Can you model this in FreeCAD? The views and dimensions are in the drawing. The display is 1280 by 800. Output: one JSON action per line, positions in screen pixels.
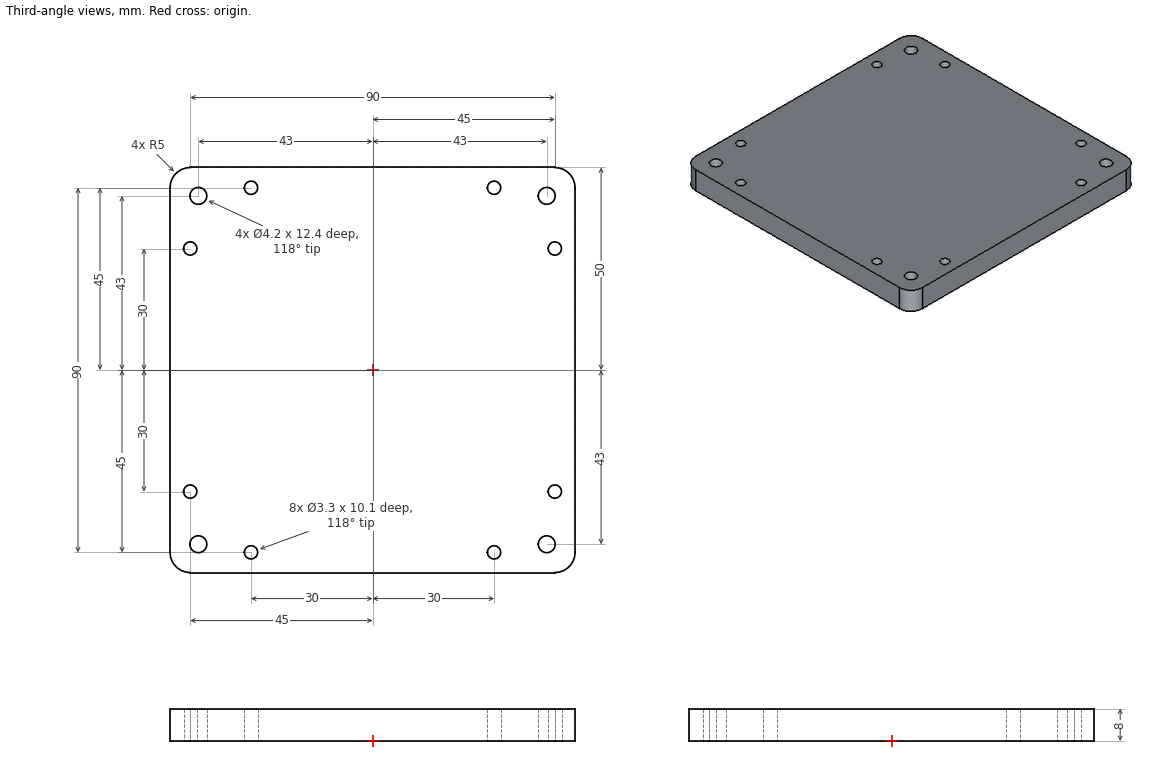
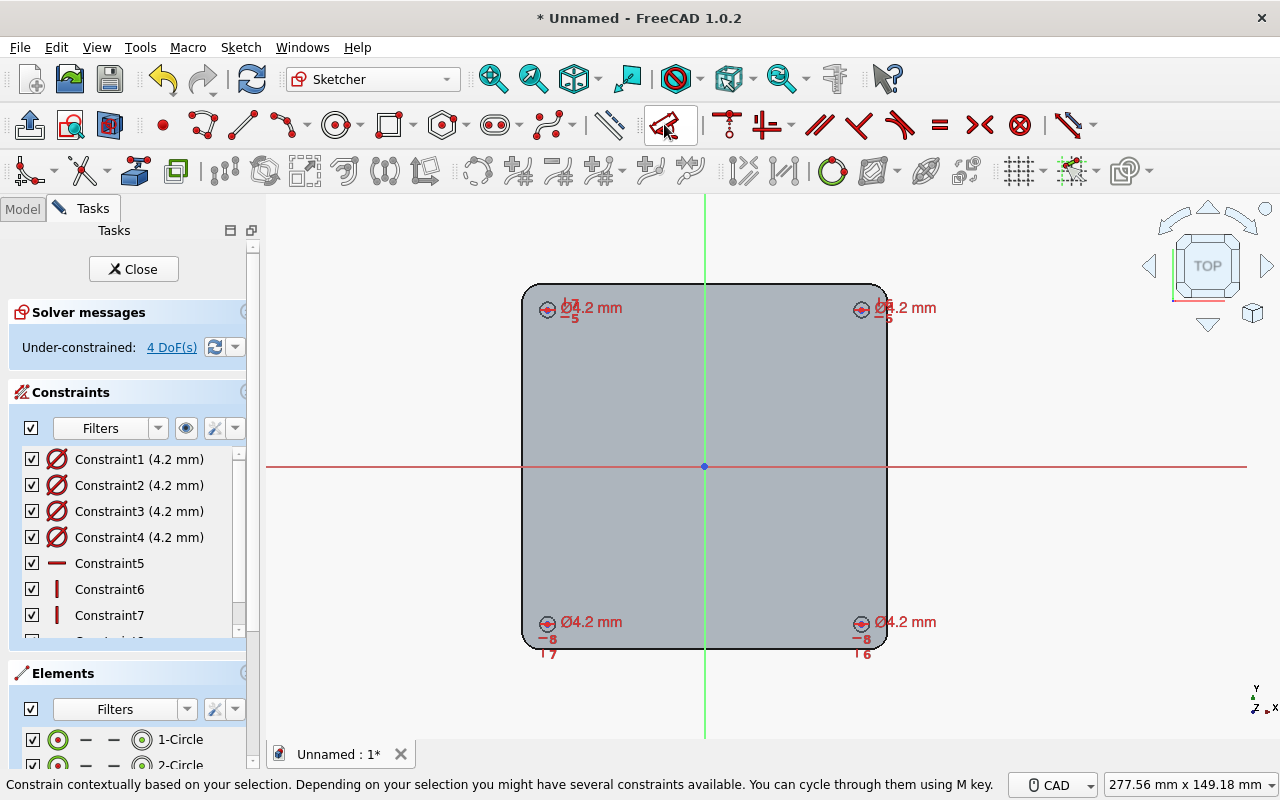
{"action": "left_click", "coordinate": [548, 310]}
{"action": "left_click", "coordinate": [626, 276]}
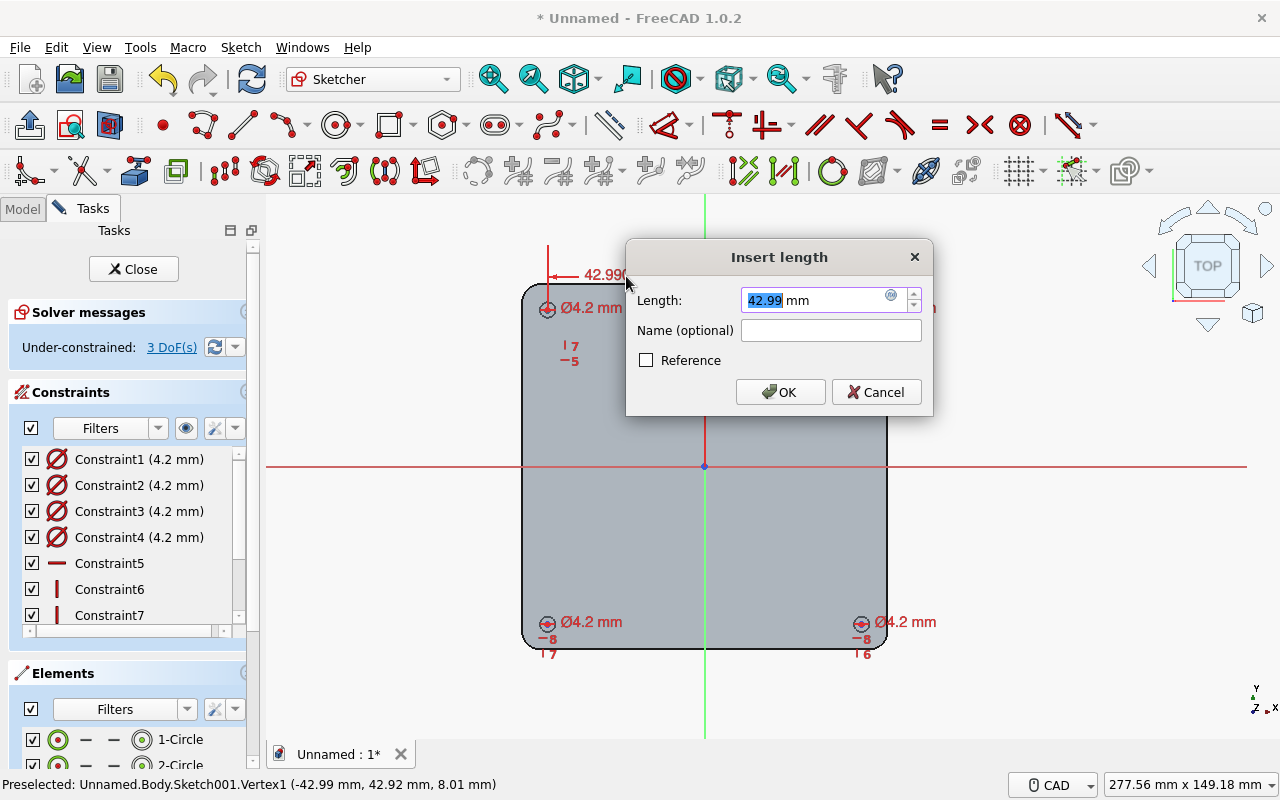
{"action": "type", "text": "43"}
{"action": "key", "text": "Return"}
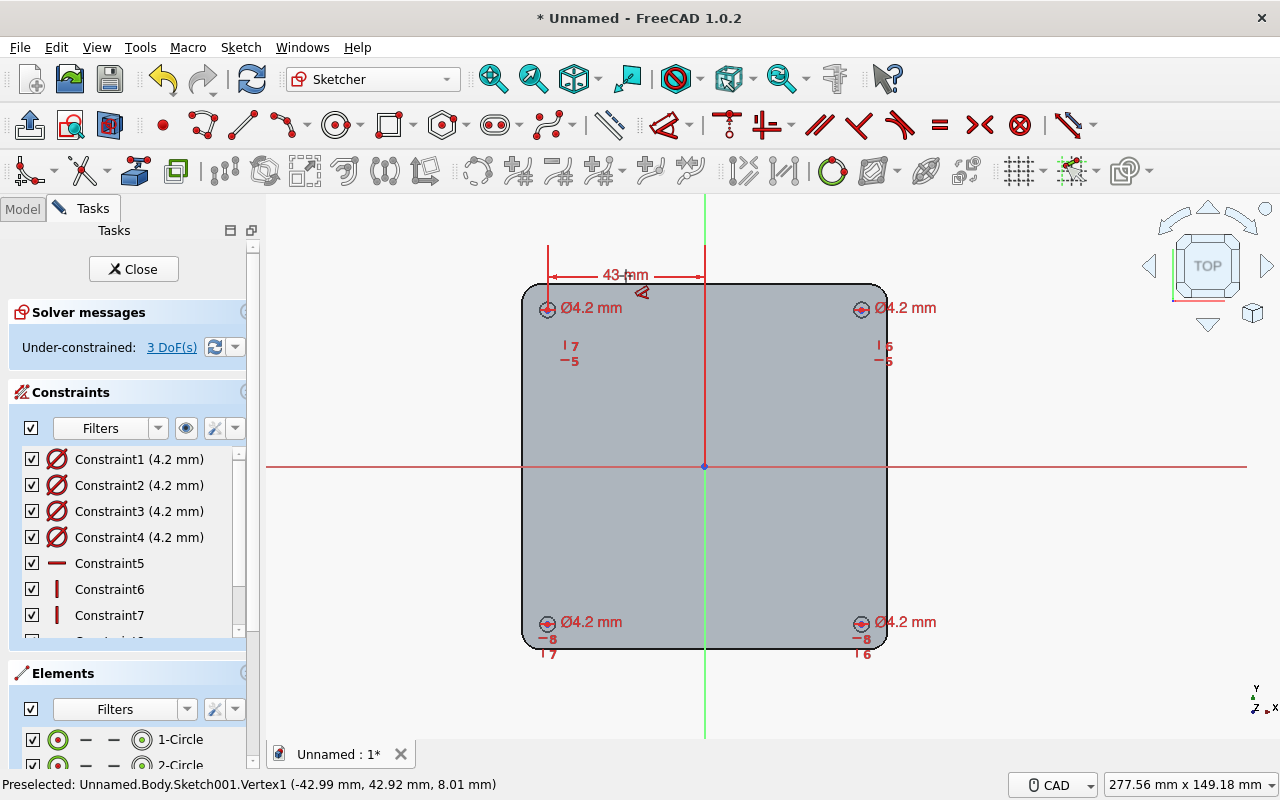
{"action": "left_click", "coordinate": [548, 310]}
{"action": "left_click", "coordinate": [514, 388]}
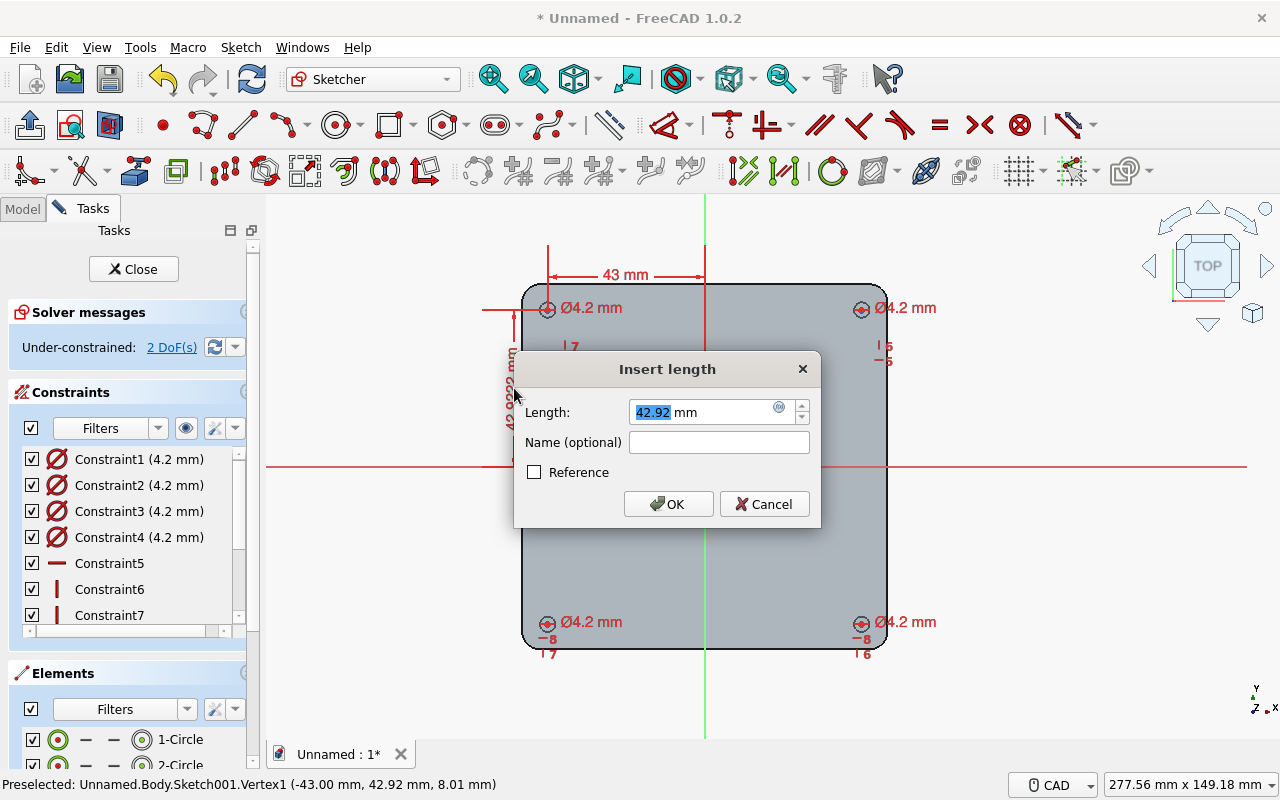
{"action": "type", "text": "43"}
{"action": "key", "text": "Return"}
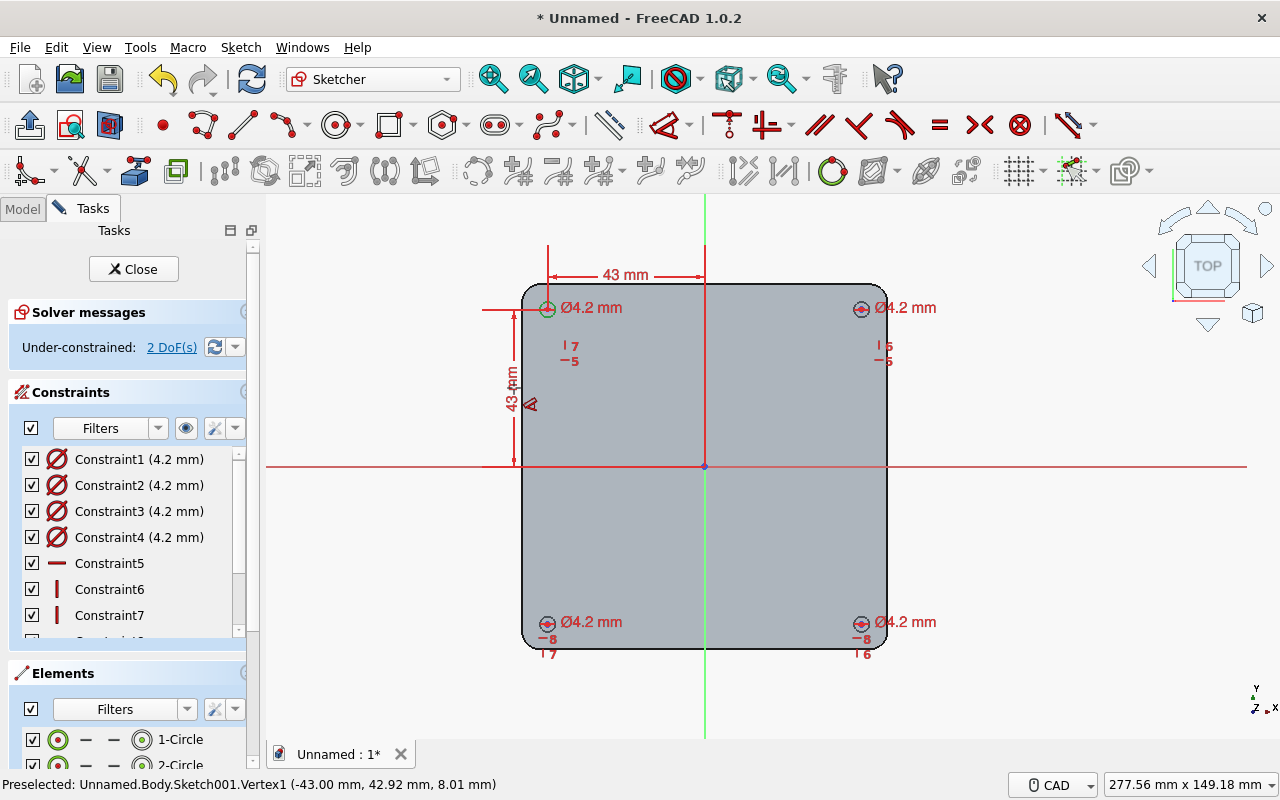
{"action": "left_click", "coordinate": [862, 310]}
{"action": "left_click", "coordinate": [783, 276]}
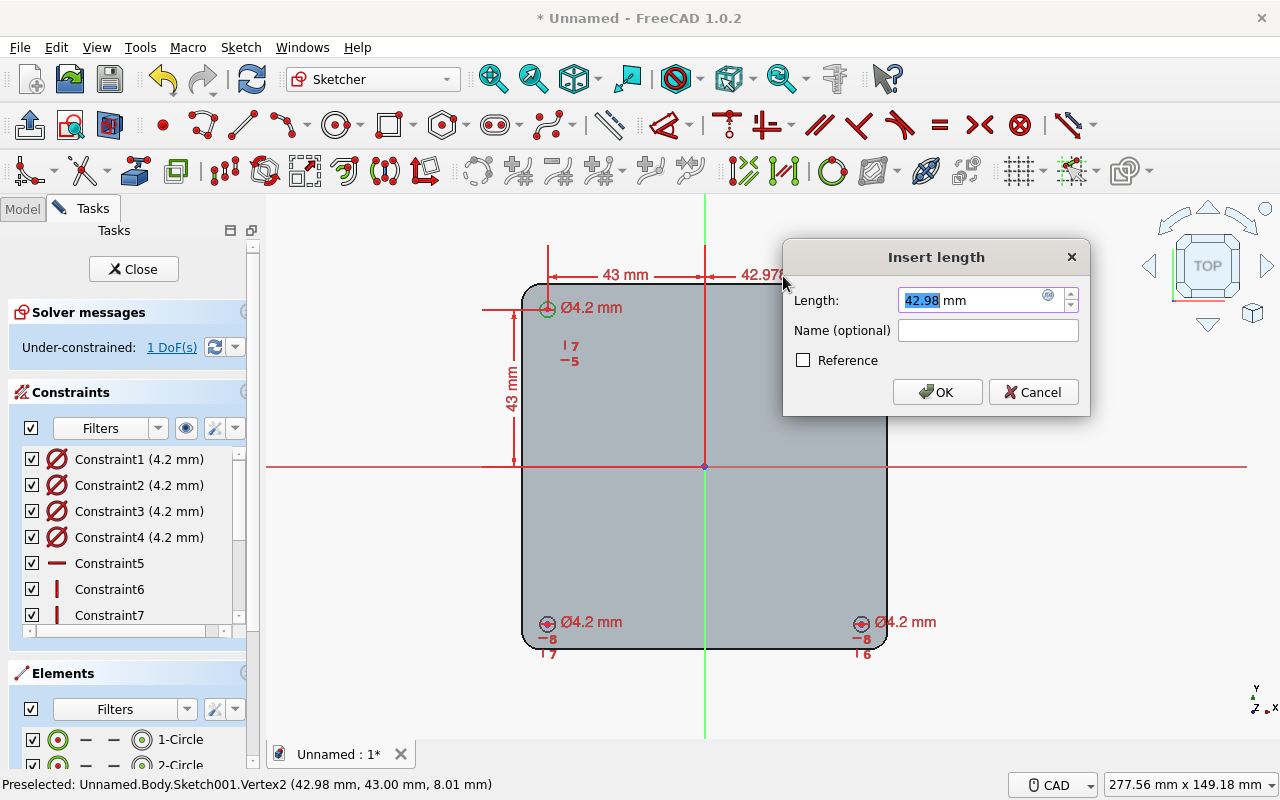
{"action": "type", "text": "43"}
{"action": "key", "text": "Return"}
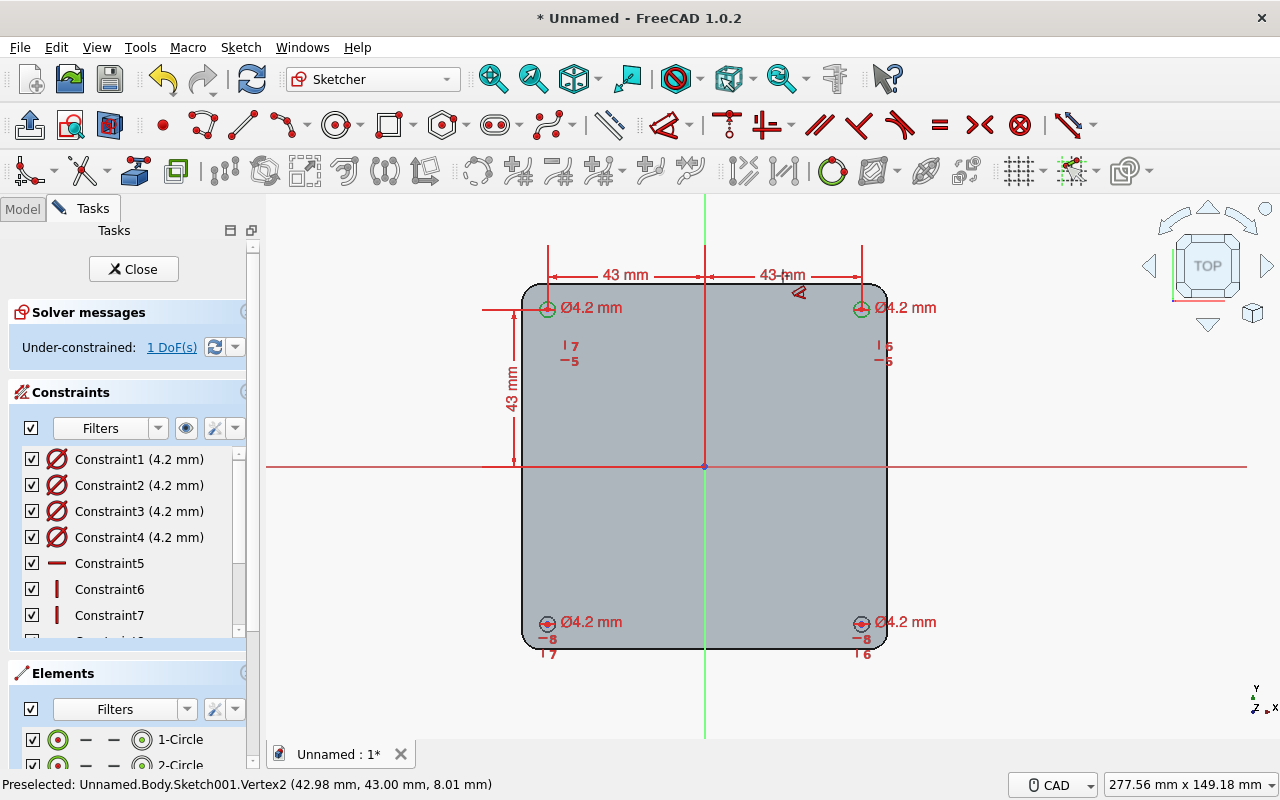
{"action": "left_click", "coordinate": [862, 624]}
{"action": "left_click", "coordinate": [896, 546]}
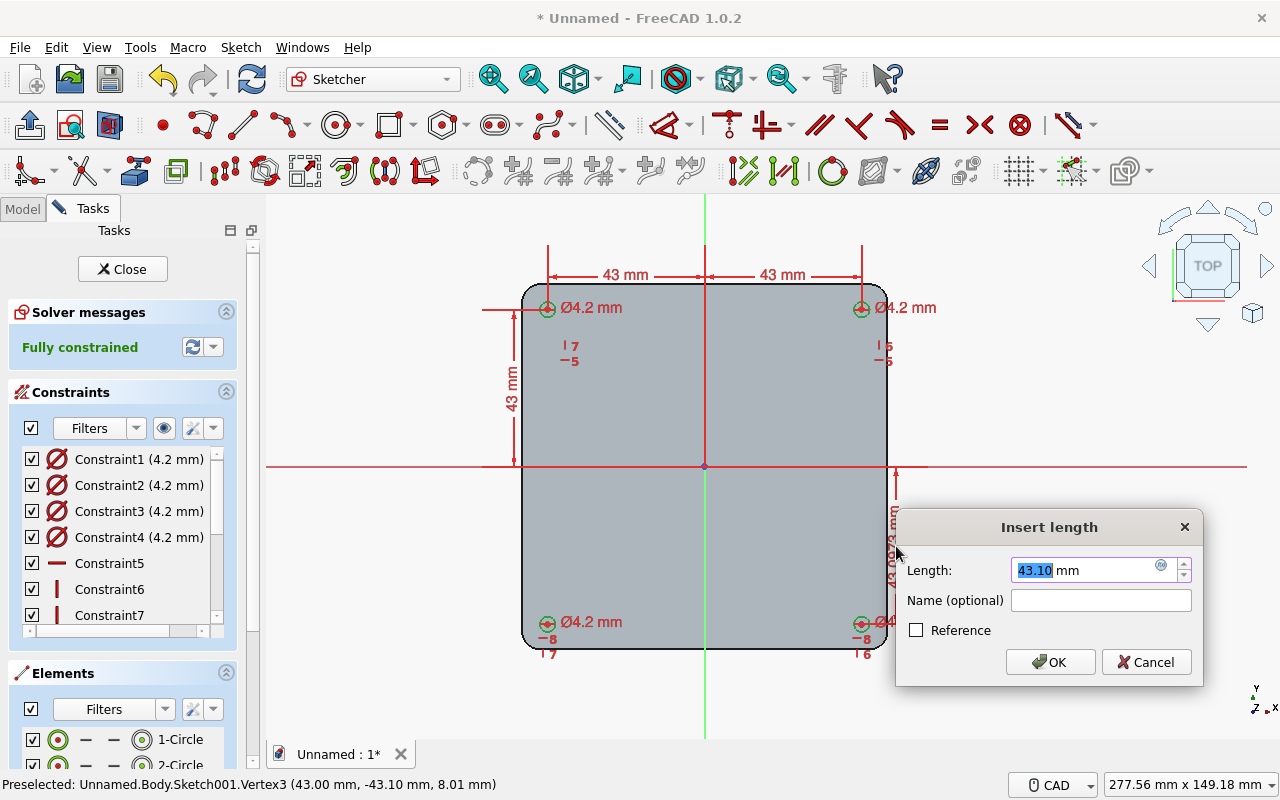
{"action": "type", "text": "43"}
{"action": "key", "text": "Return"}
{"action": "key", "text": "Escape"}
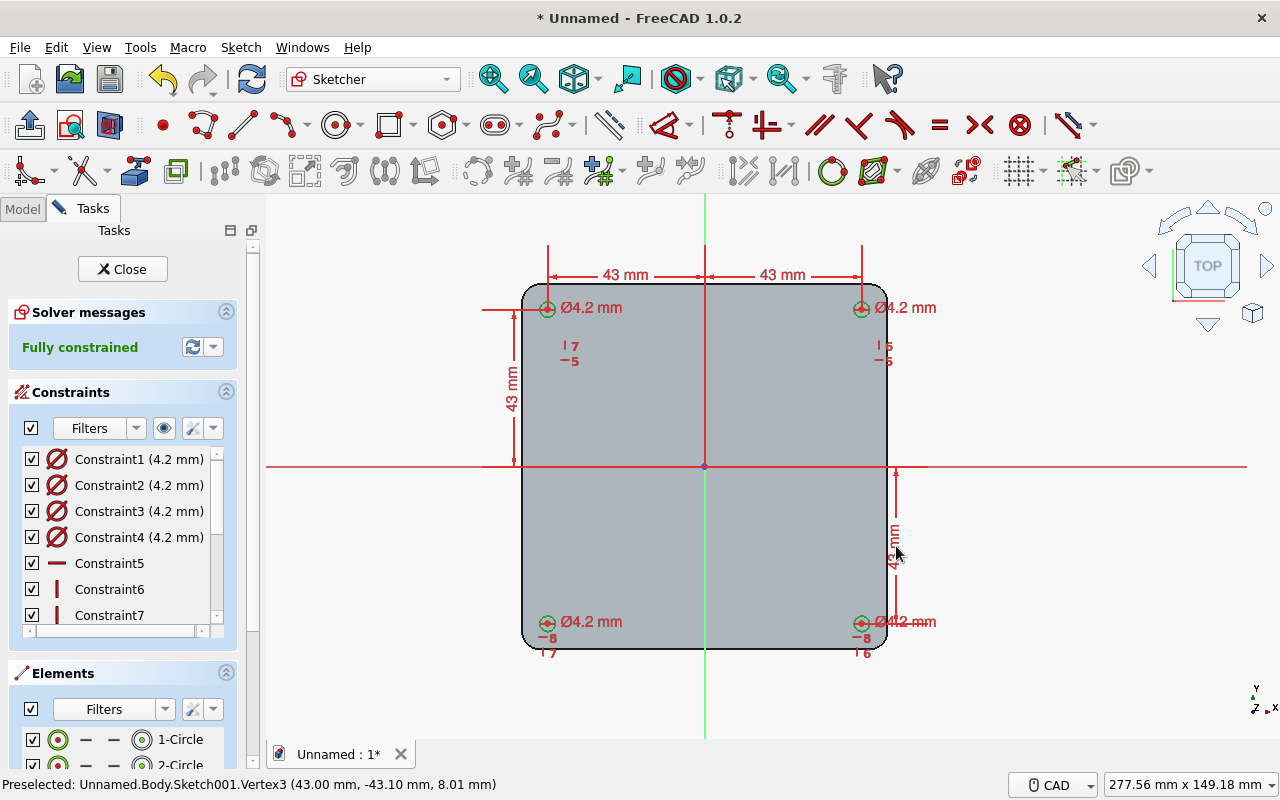
{"action": "left_click", "coordinate": [123, 269]}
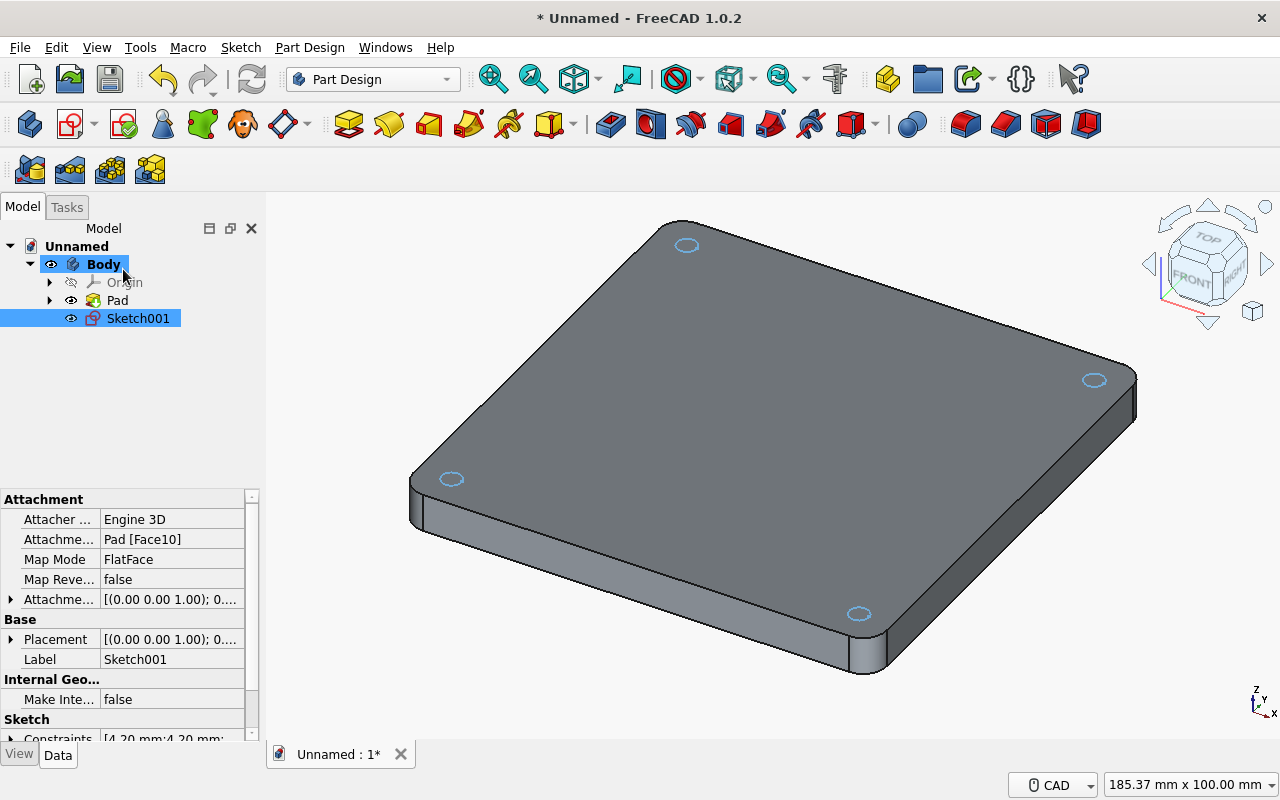
{"action": "left_click", "coordinate": [652, 124]}